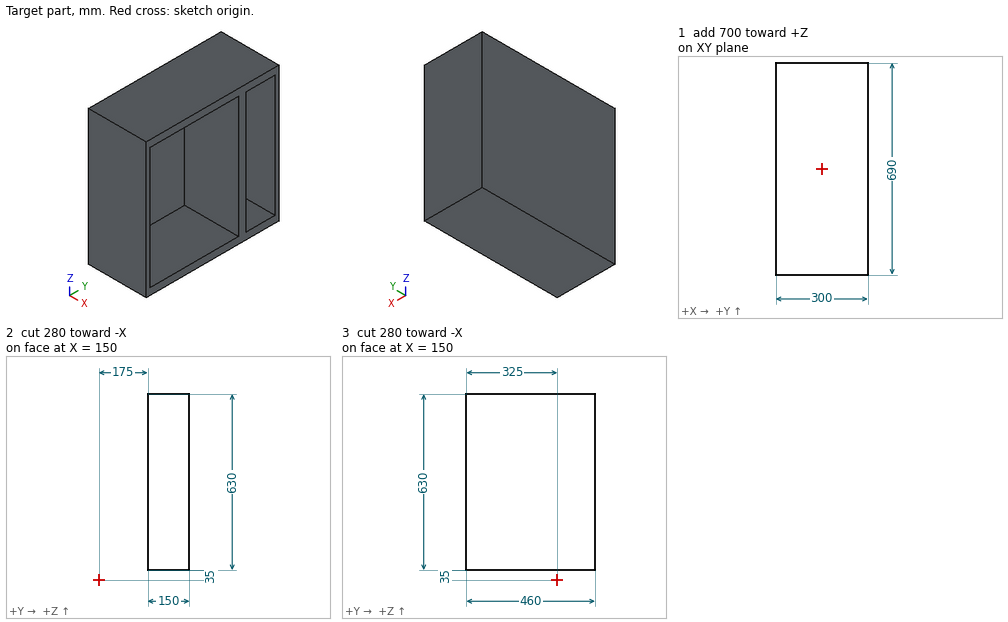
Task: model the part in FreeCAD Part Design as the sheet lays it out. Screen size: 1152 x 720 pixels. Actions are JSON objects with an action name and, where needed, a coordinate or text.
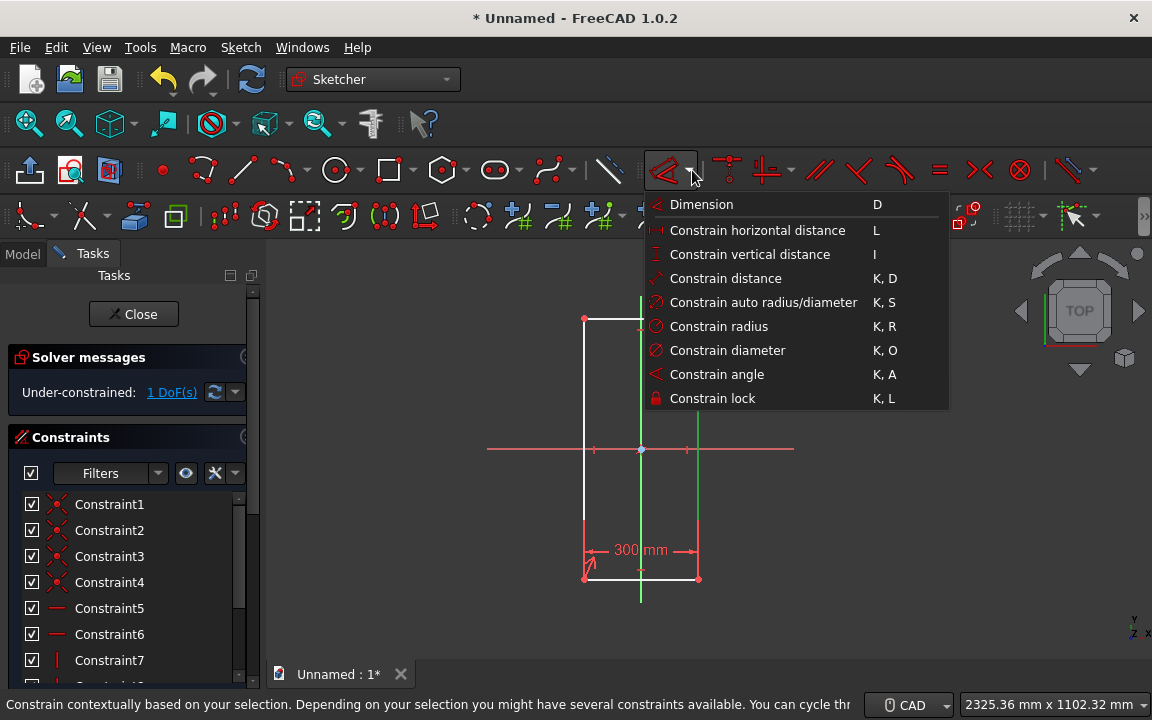
{"action": "left_click", "coordinate": [797, 254]}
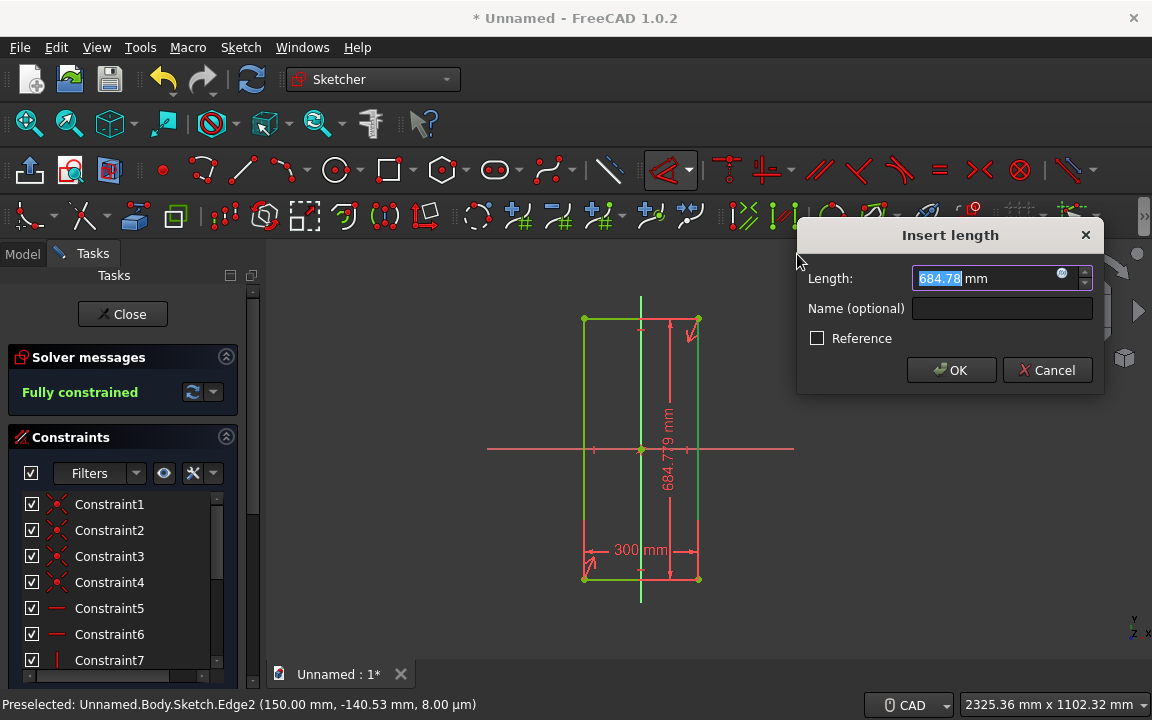
{"action": "type", "text": "690"}
{"action": "key", "text": "Return"}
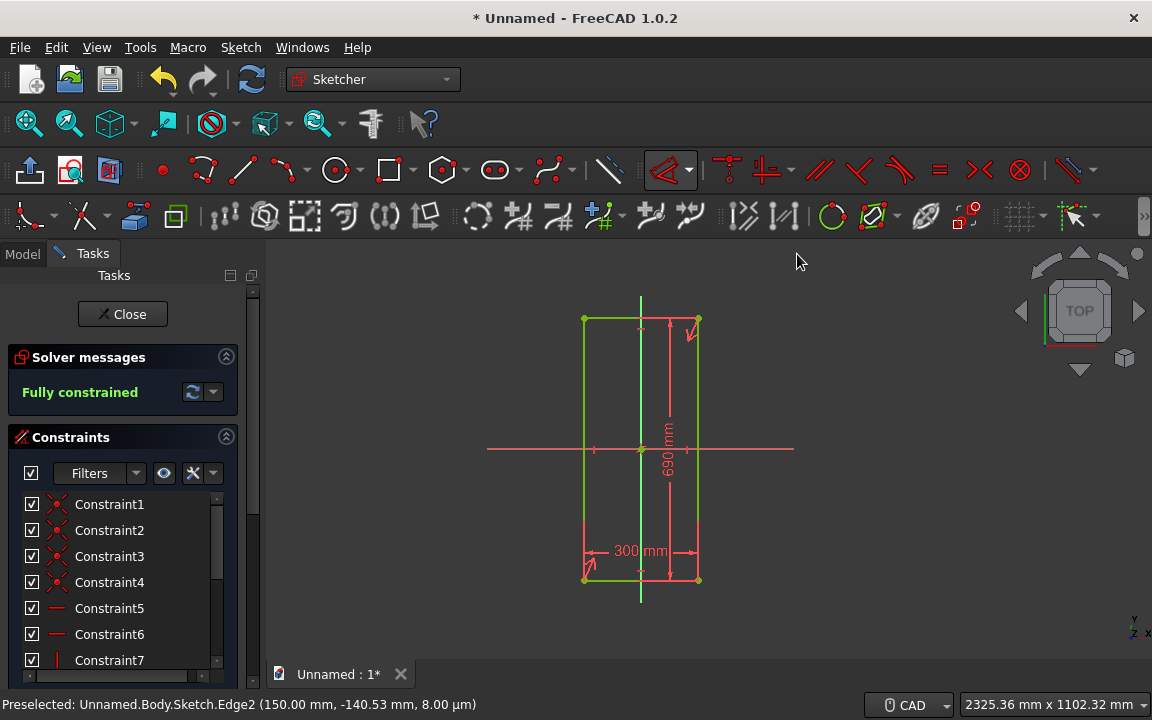
{"action": "left_click", "coordinate": [123, 314]}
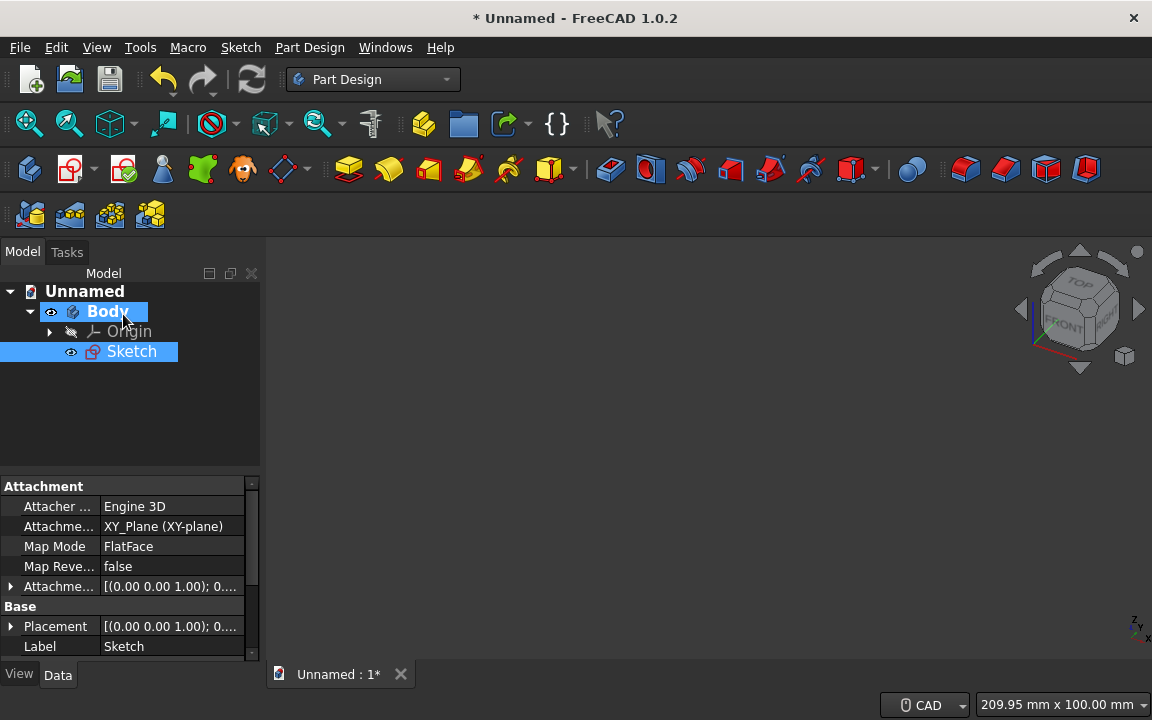
{"action": "left_click", "coordinate": [350, 170]}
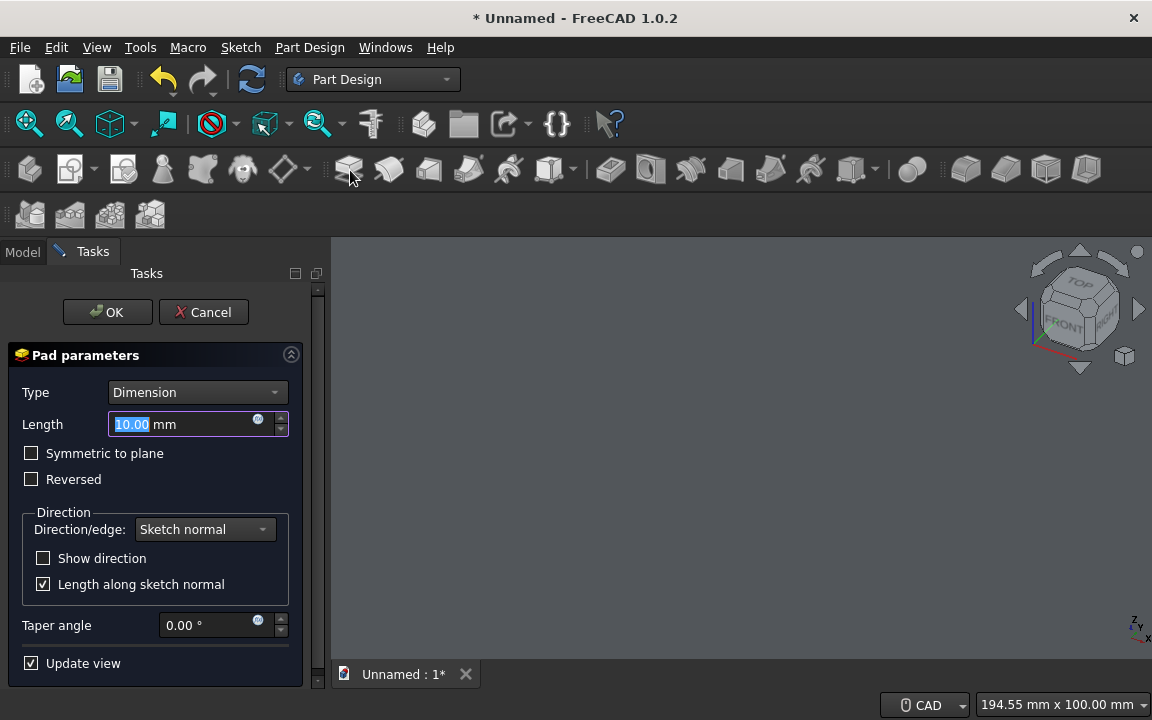
{"action": "type", "text": "700"}
{"action": "key", "text": "Tab"}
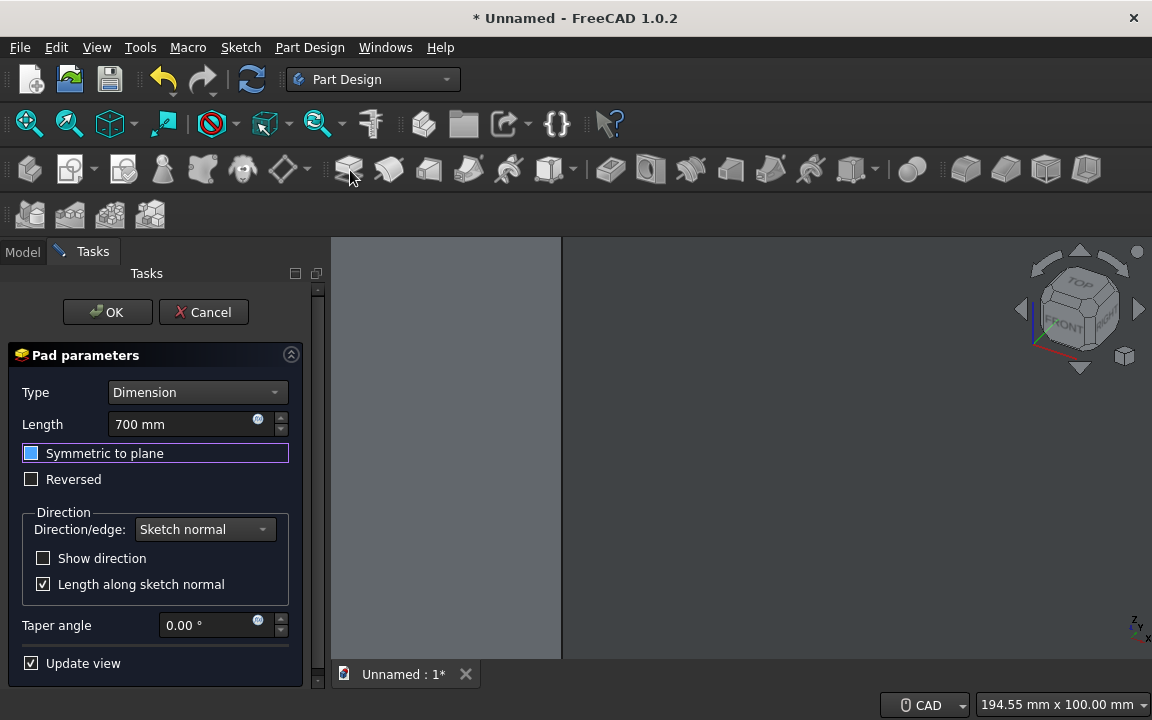
{"action": "left_click", "coordinate": [108, 312]}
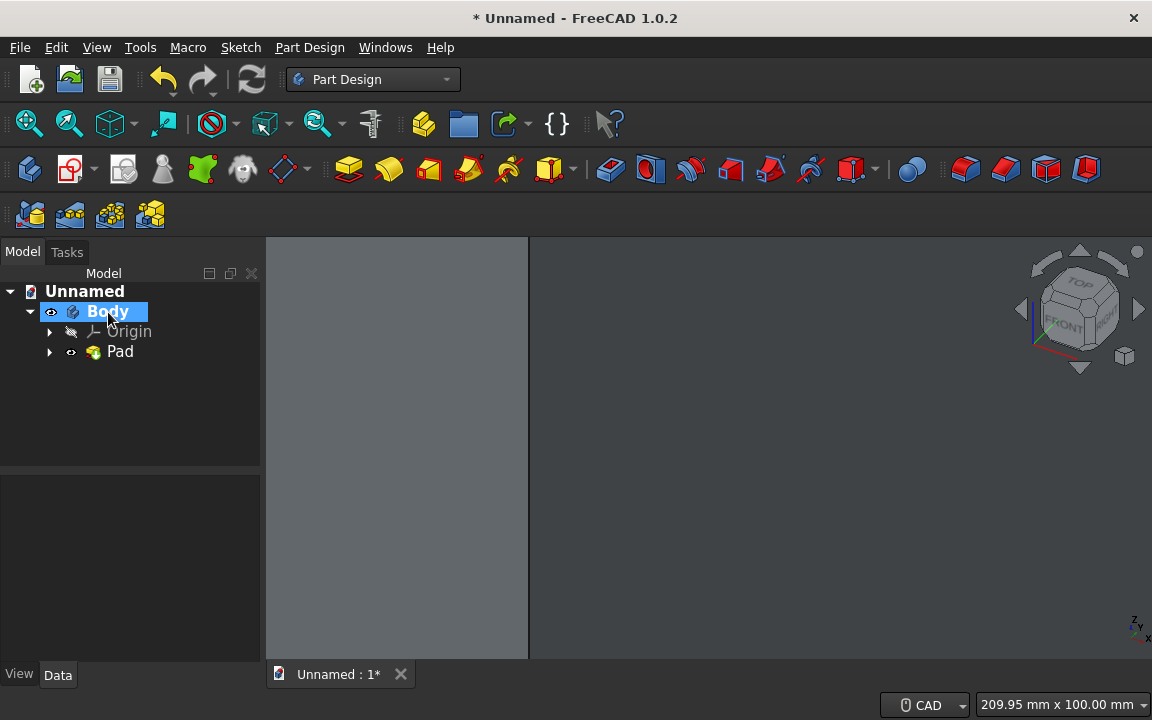
{"action": "left_click", "coordinate": [30, 124]}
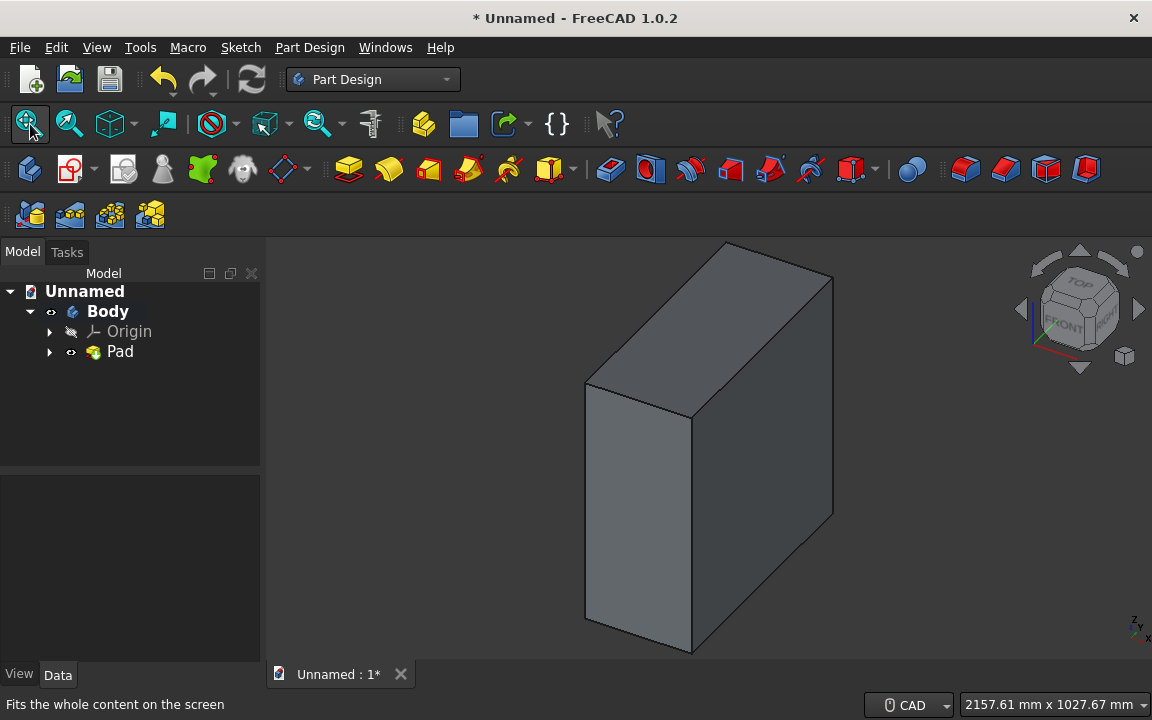
{"action": "left_click", "coordinate": [762, 465]}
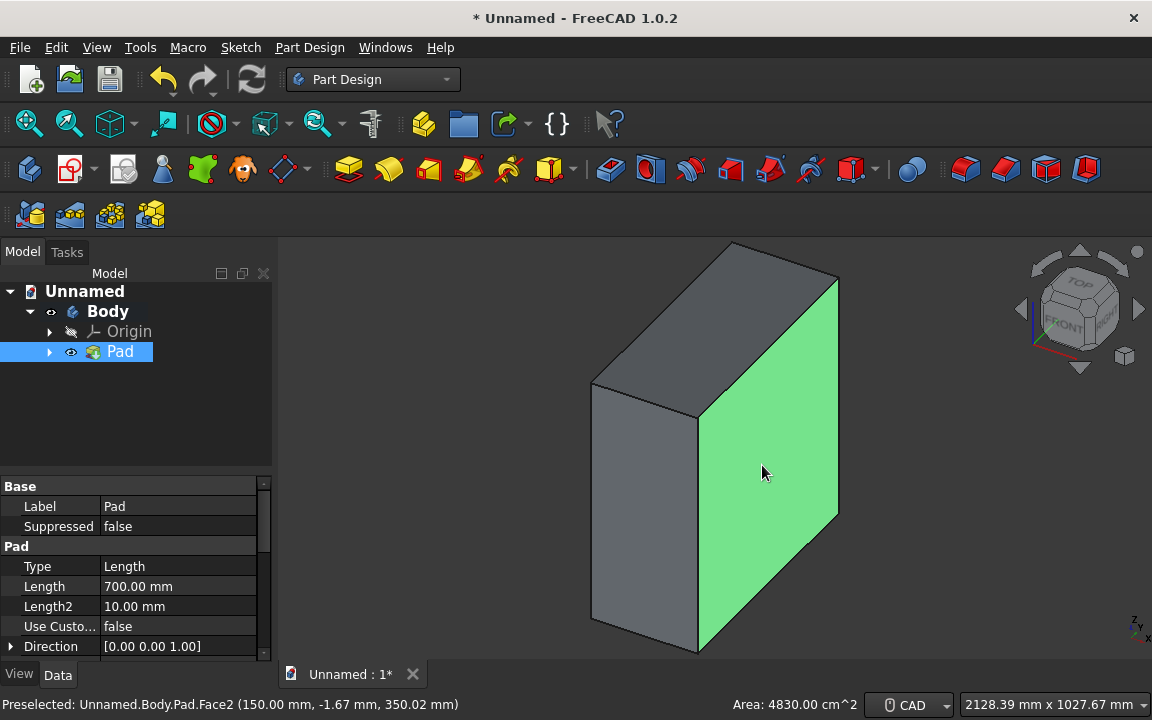
{"action": "left_click", "coordinate": [70, 170]}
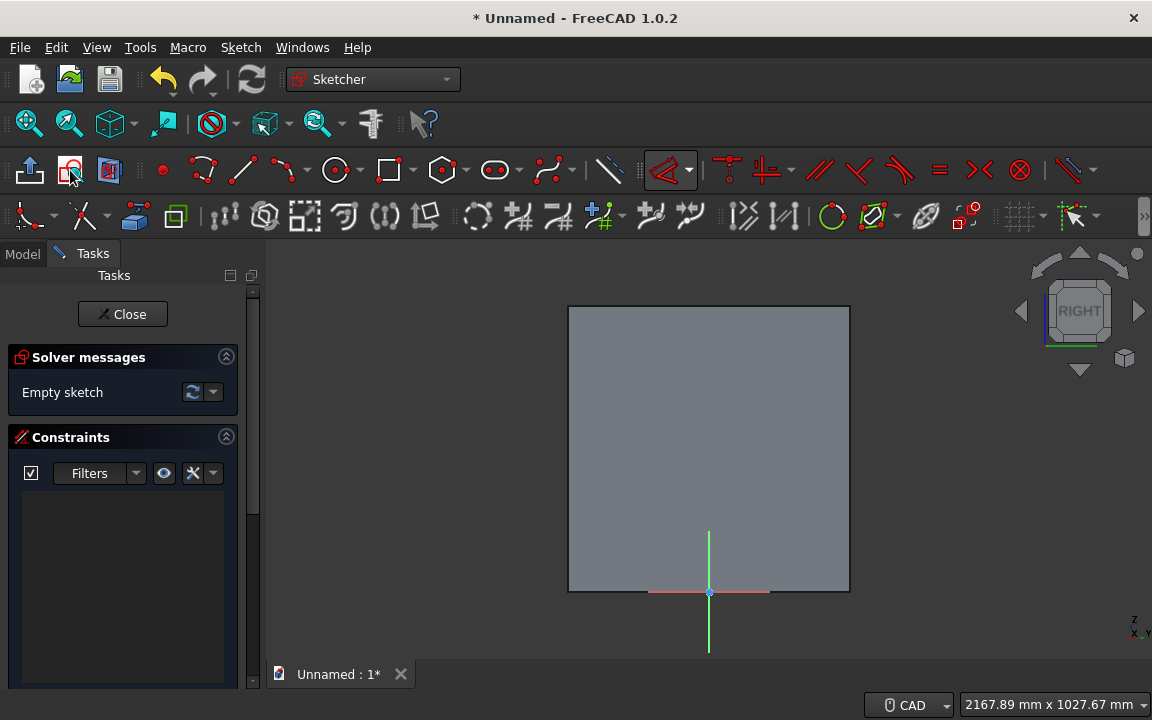
{"action": "key", "text": "g r"}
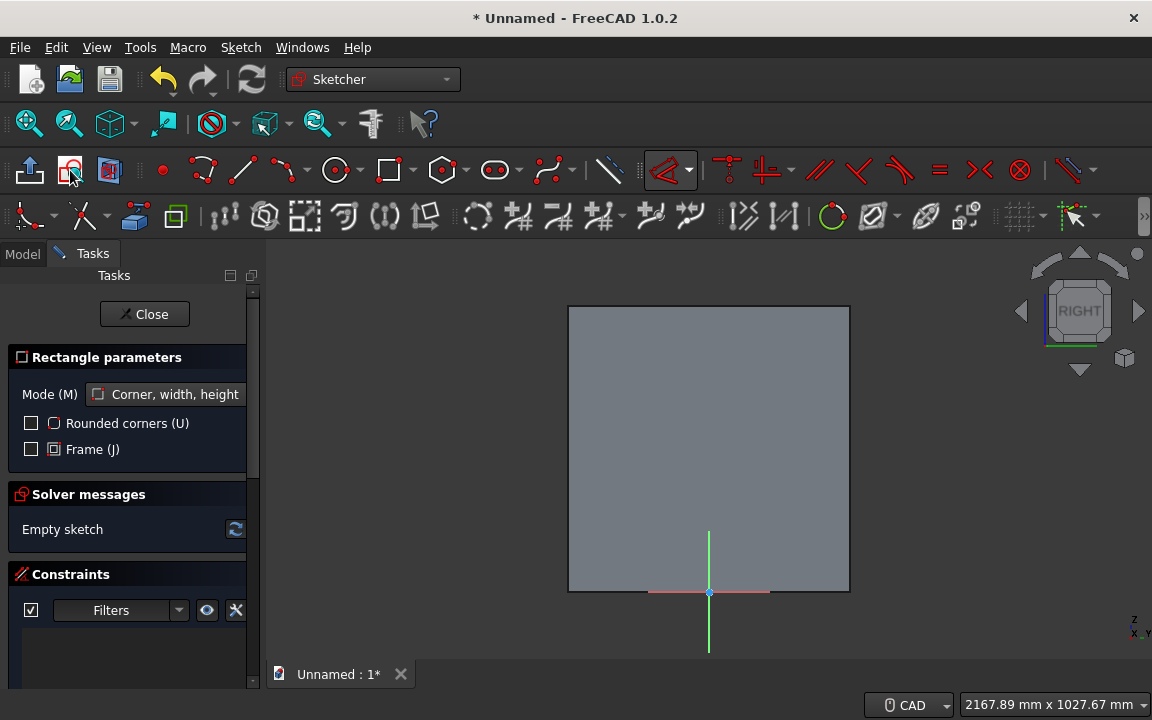
{"action": "left_click", "coordinate": [781, 320]}
{"action": "left_click", "coordinate": [842, 578]}
{"action": "key", "text": "Escape"}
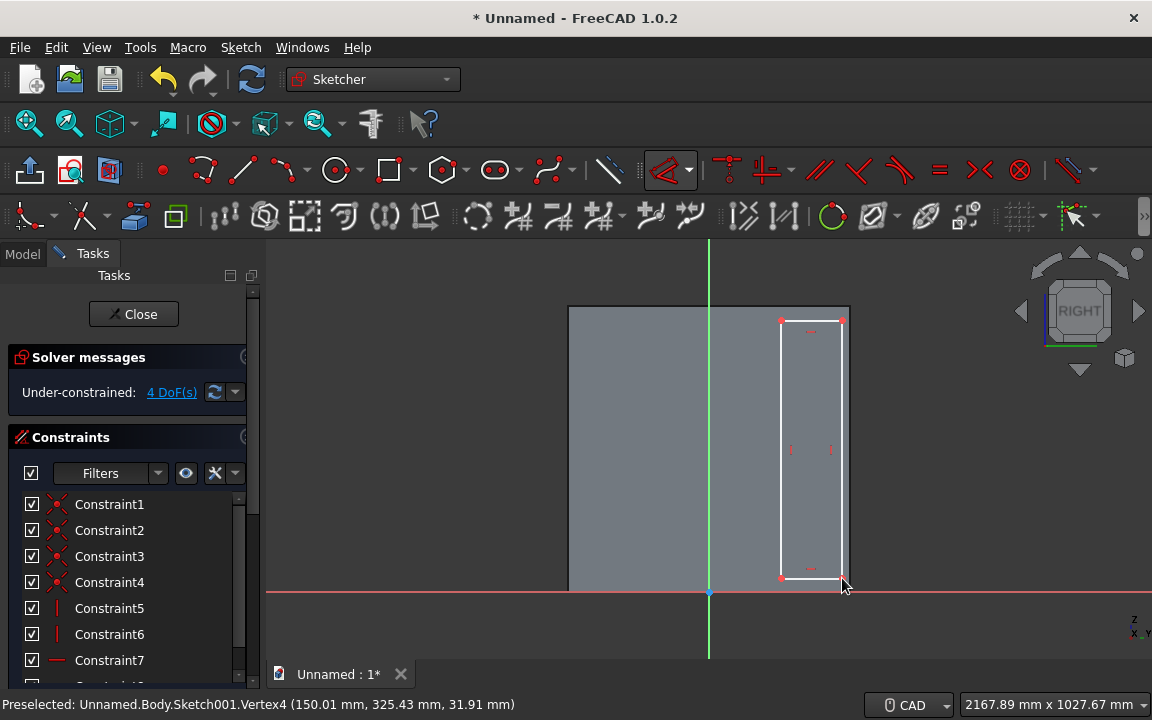
{"action": "left_click", "coordinate": [781, 398]}